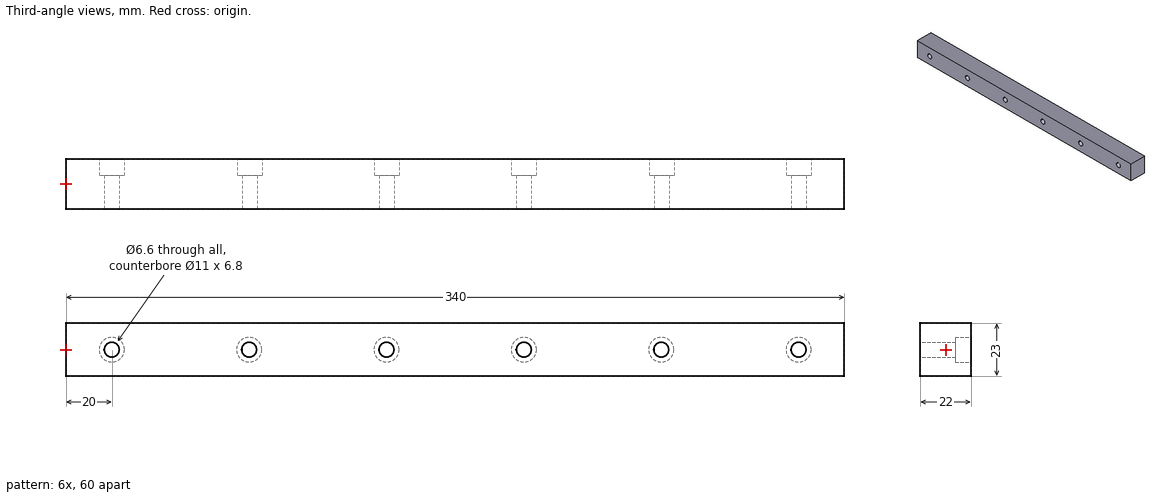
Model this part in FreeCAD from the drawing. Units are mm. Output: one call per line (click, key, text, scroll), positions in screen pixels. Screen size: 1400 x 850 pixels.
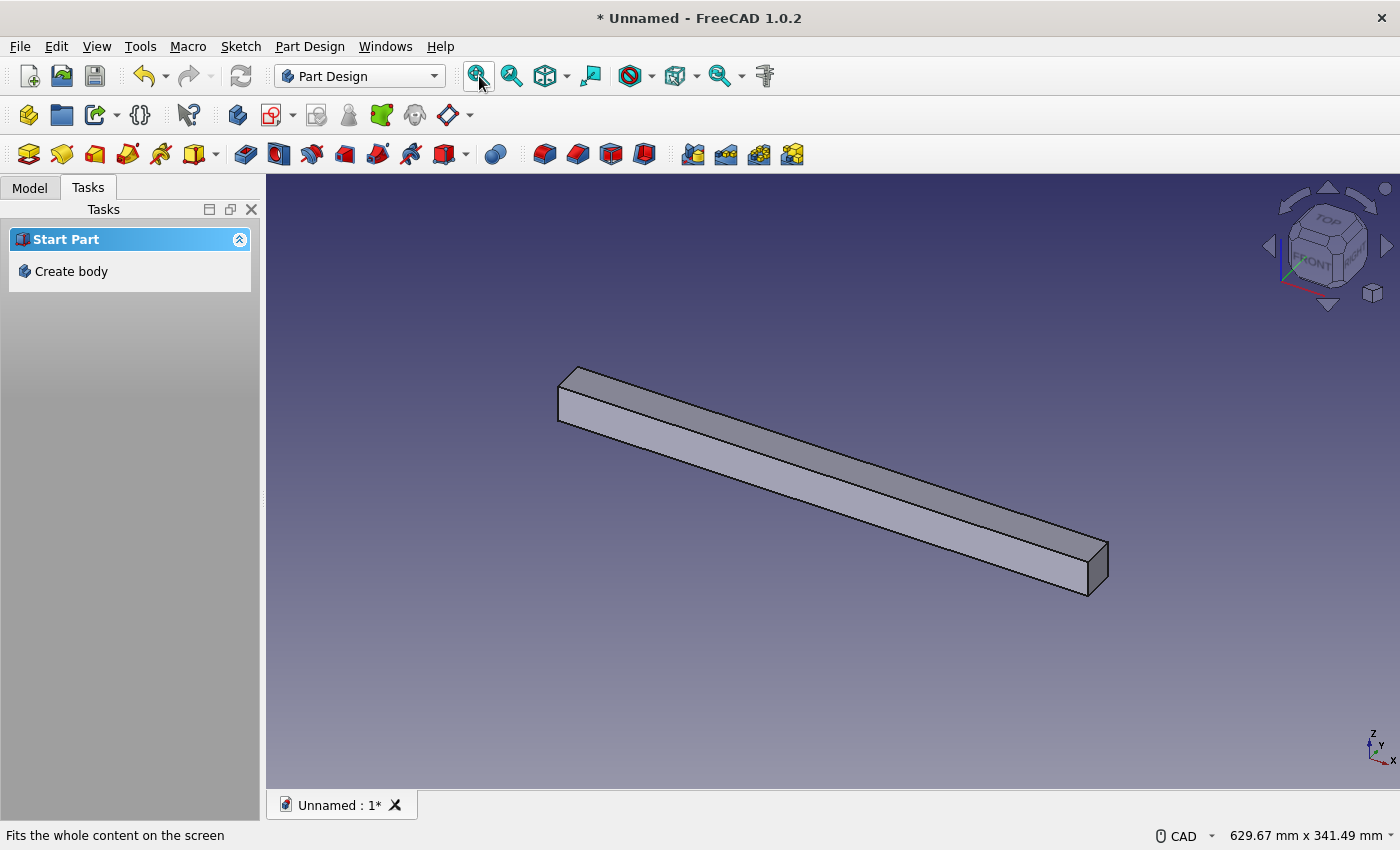
key(4)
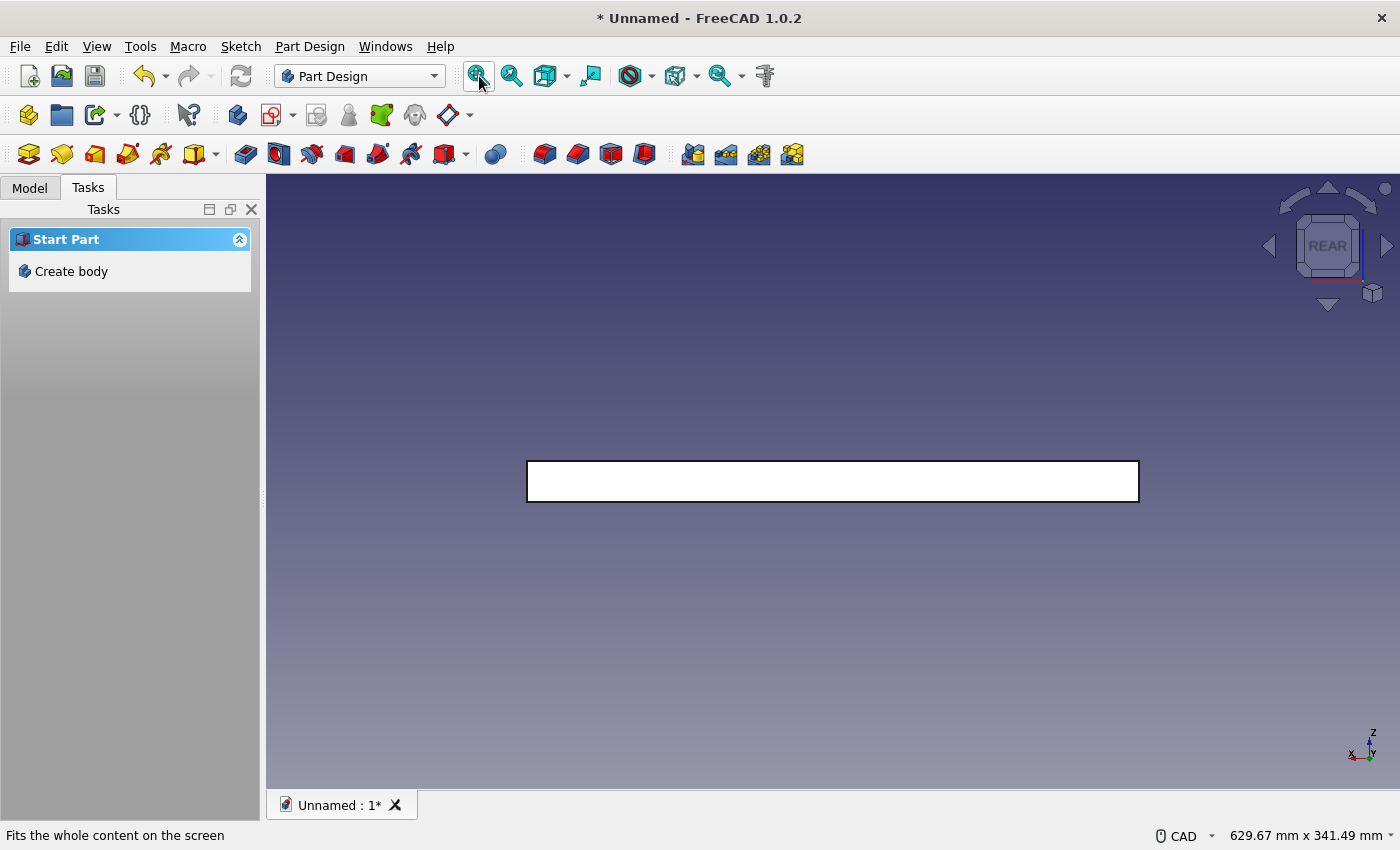
click(833, 481)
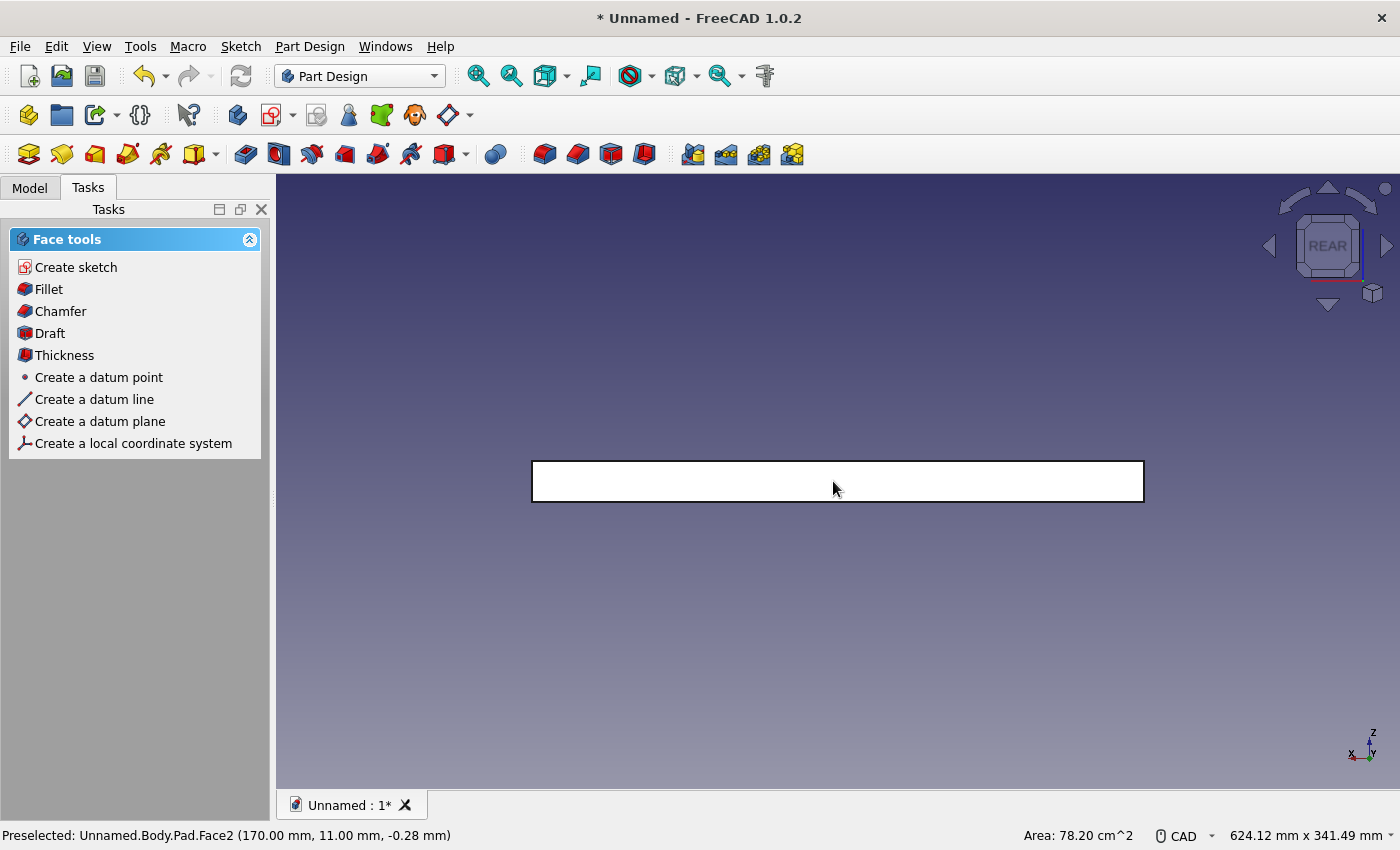
click(270, 116)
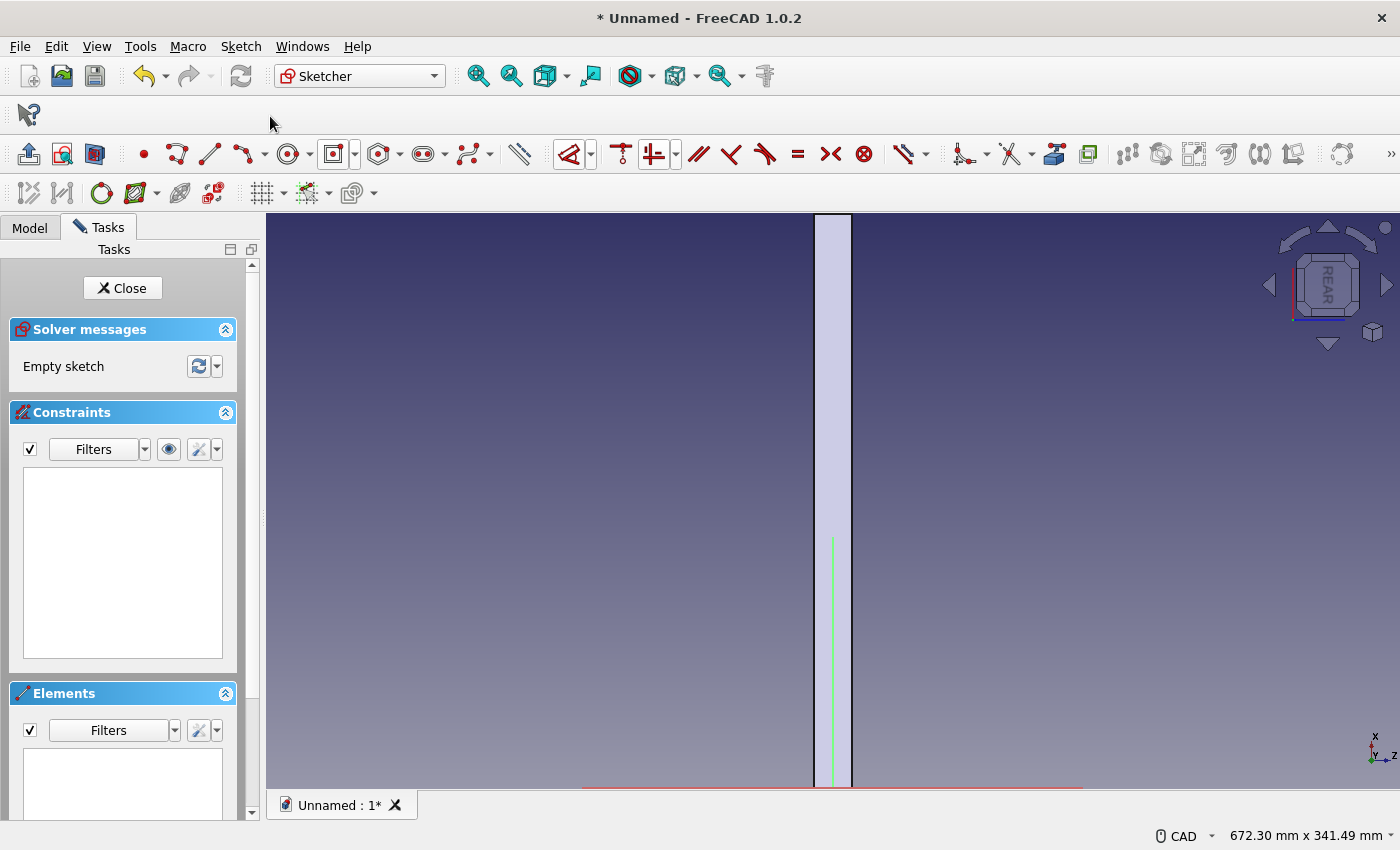
scroll(837, 761, up, 15)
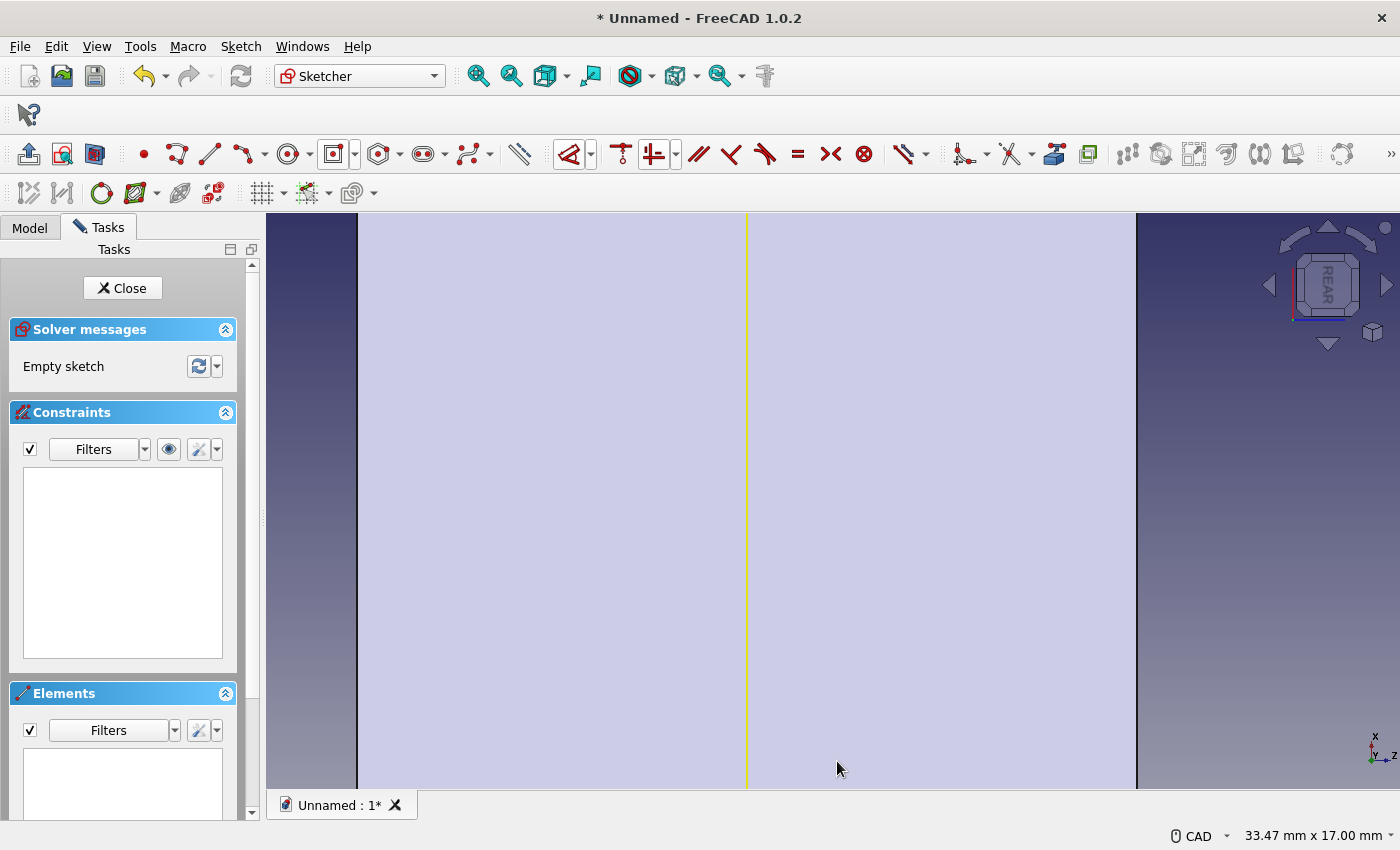
scroll(712, 761, up, 2)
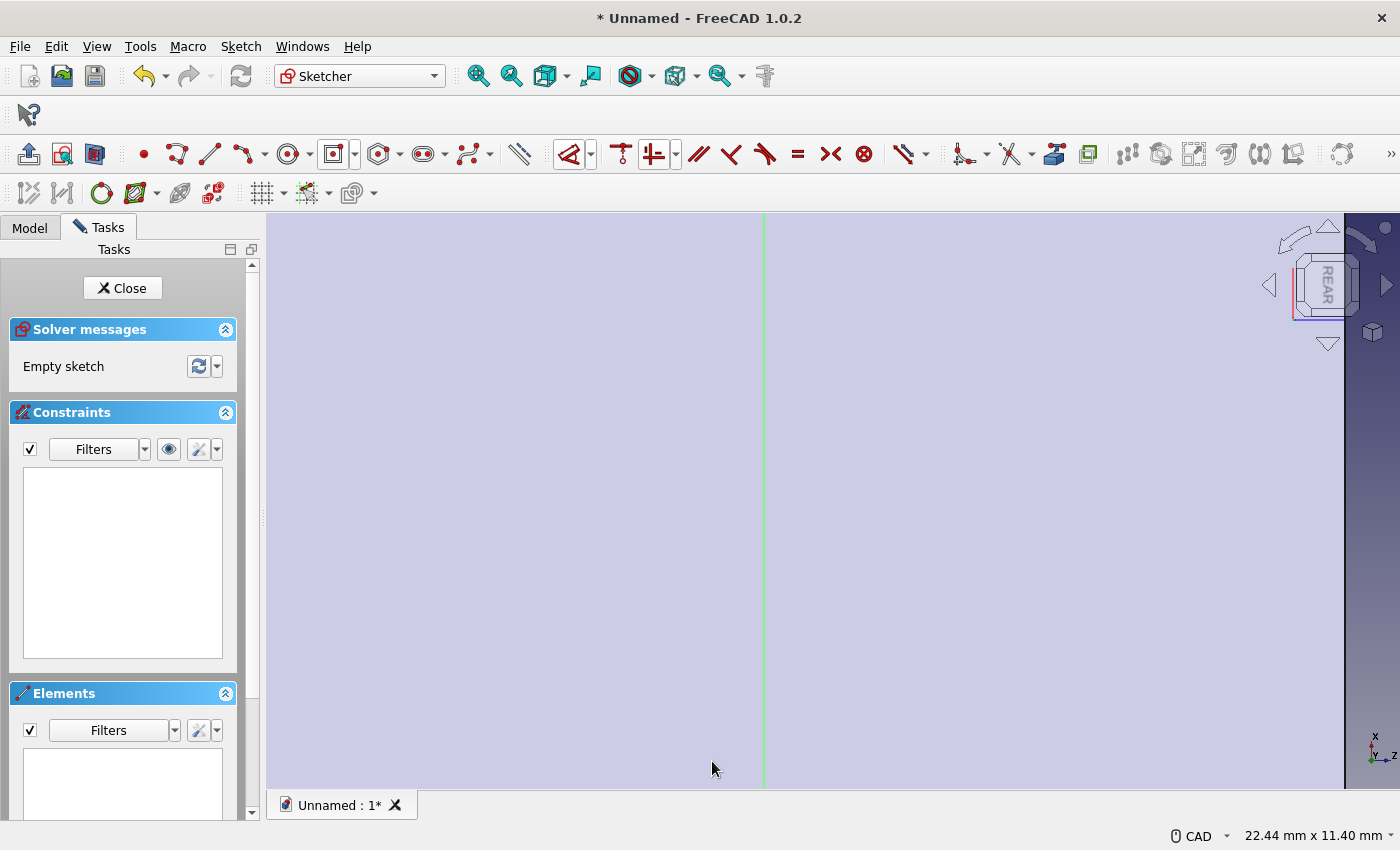
click(288, 154)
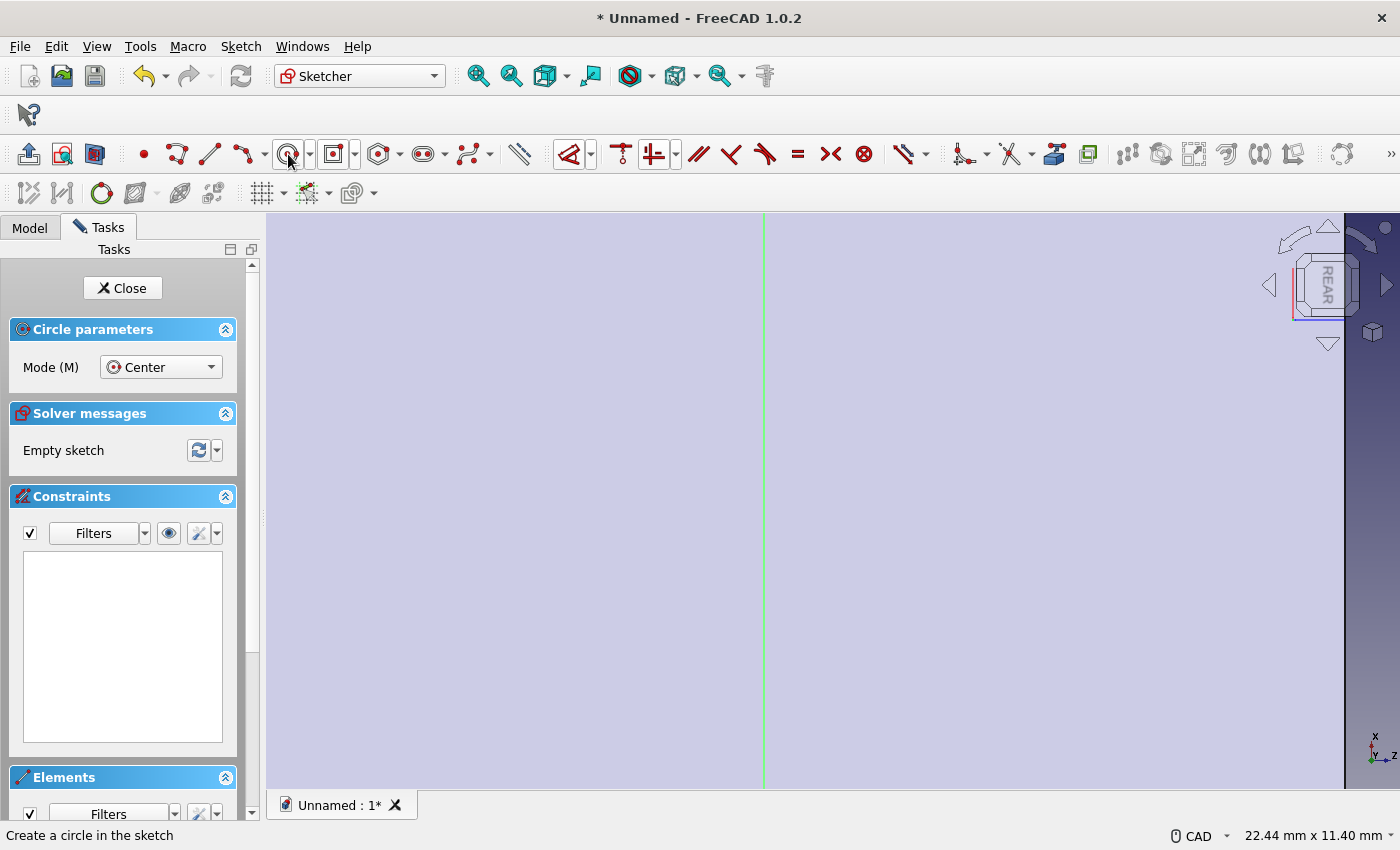
click(764, 524)
click(882, 406)
key(Escape)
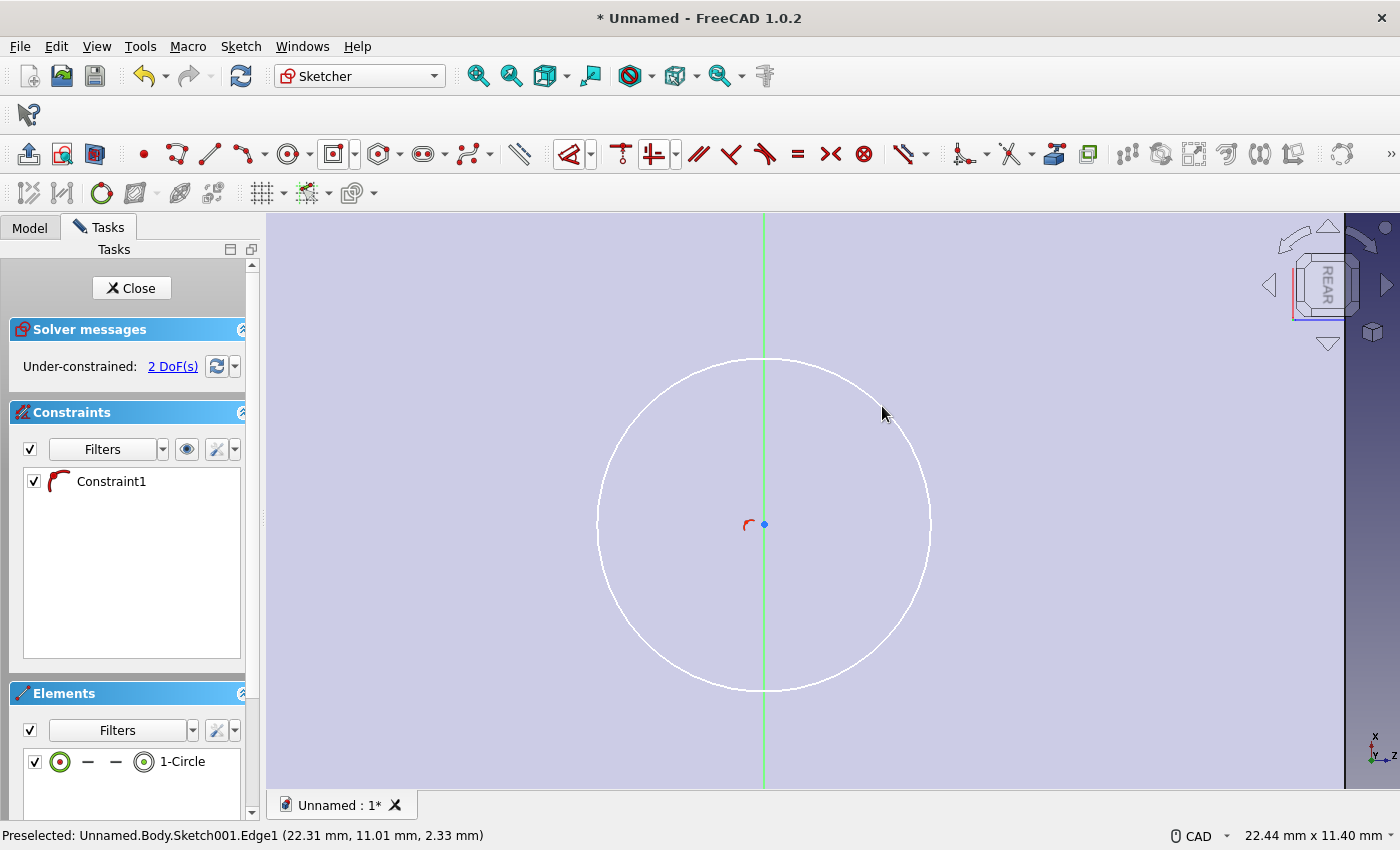
key(d)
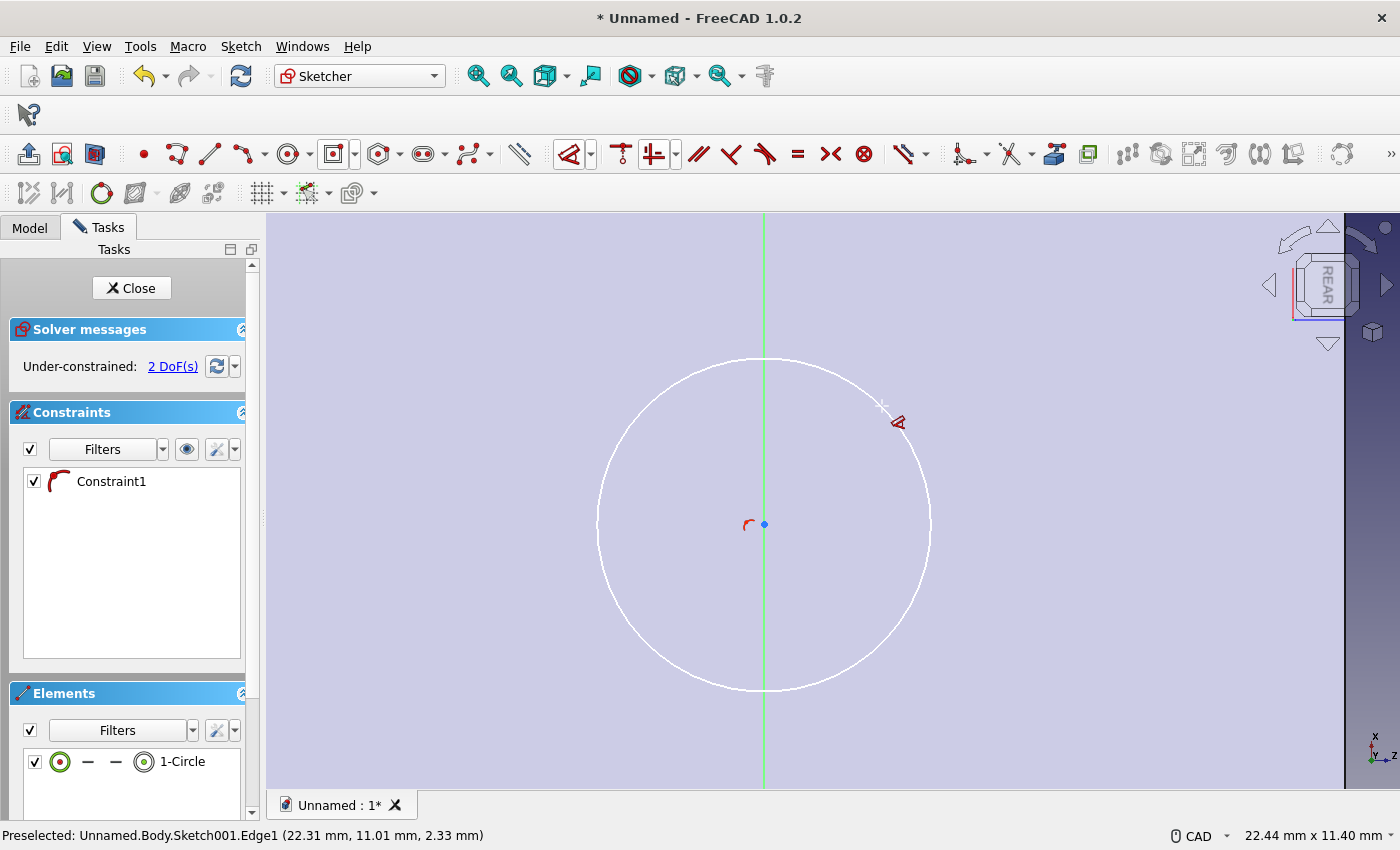
click(882, 407)
click(905, 384)